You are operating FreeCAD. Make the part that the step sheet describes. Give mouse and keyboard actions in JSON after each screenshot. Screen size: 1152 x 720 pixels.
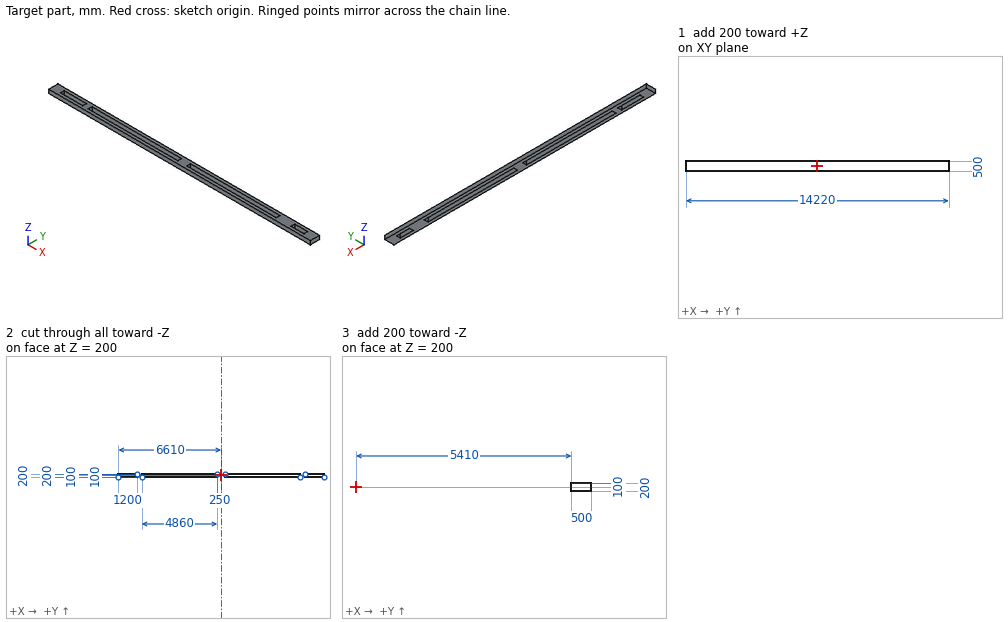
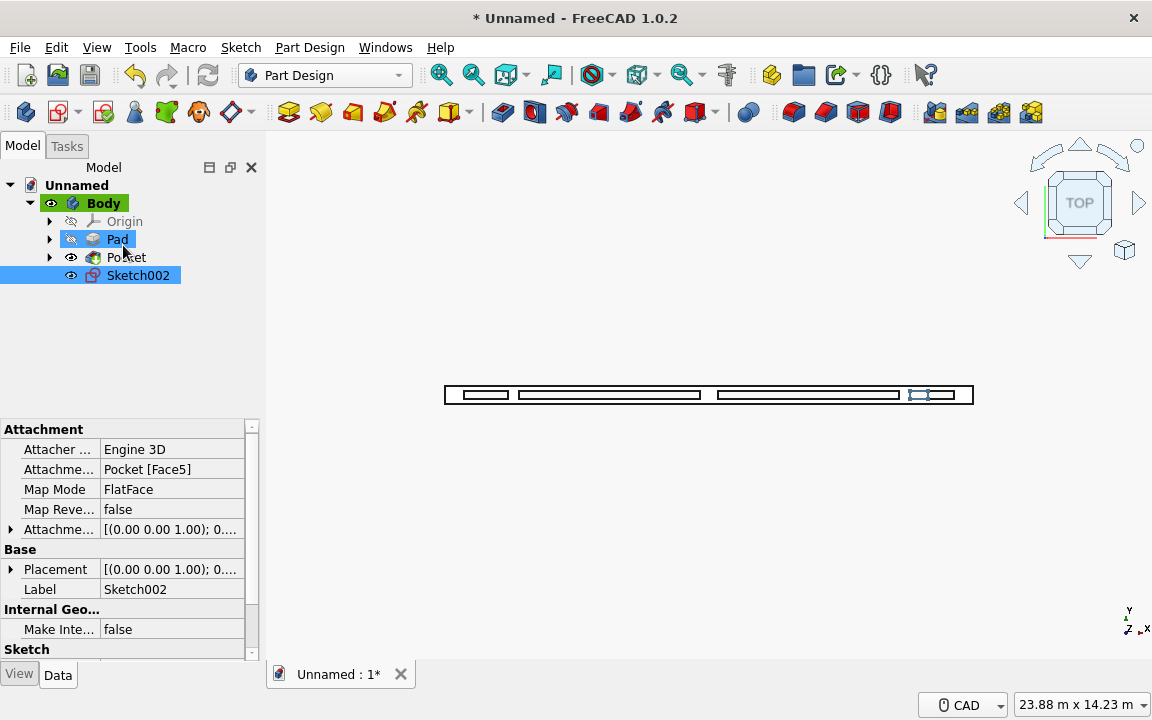
{"action": "left_click", "coordinate": [290, 112]}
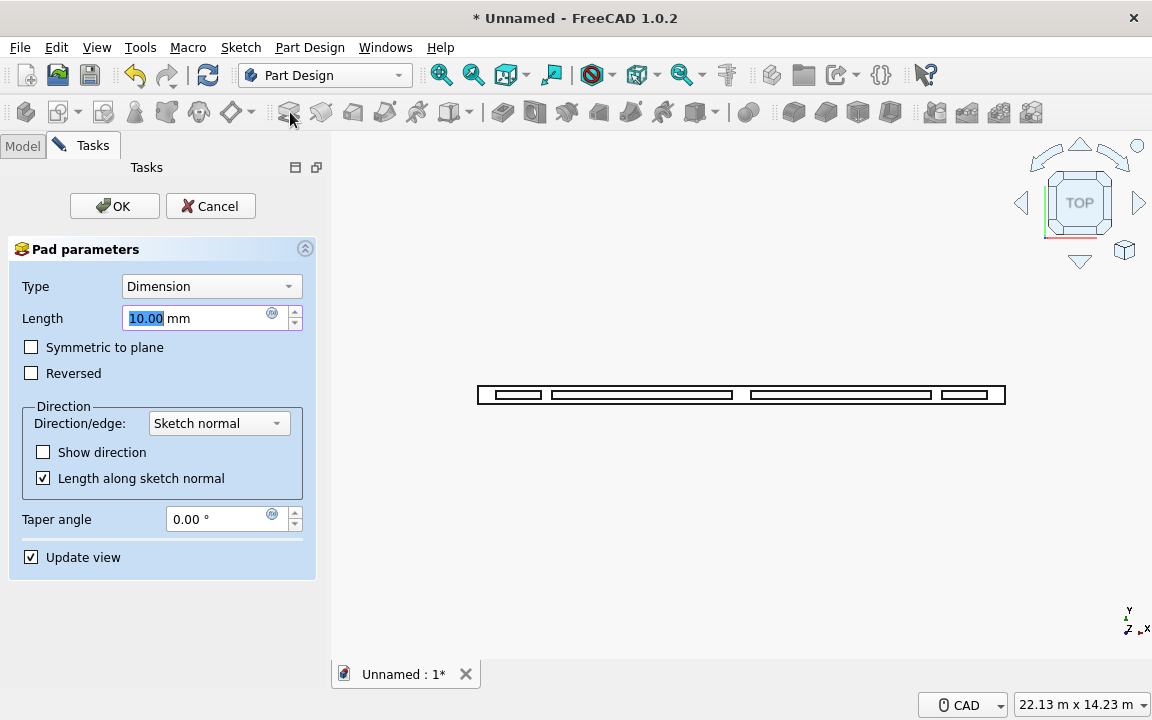
{"action": "type", "text": "200"}
{"action": "key", "text": "Tab"}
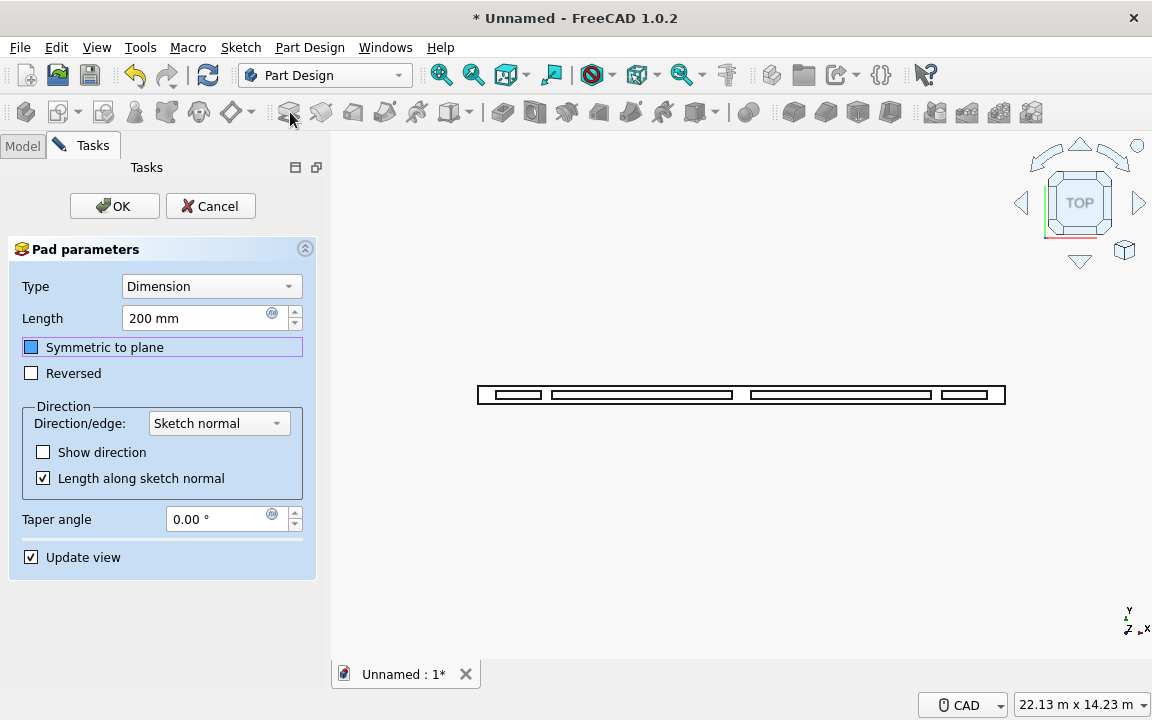
{"action": "left_click", "coordinate": [30, 373]}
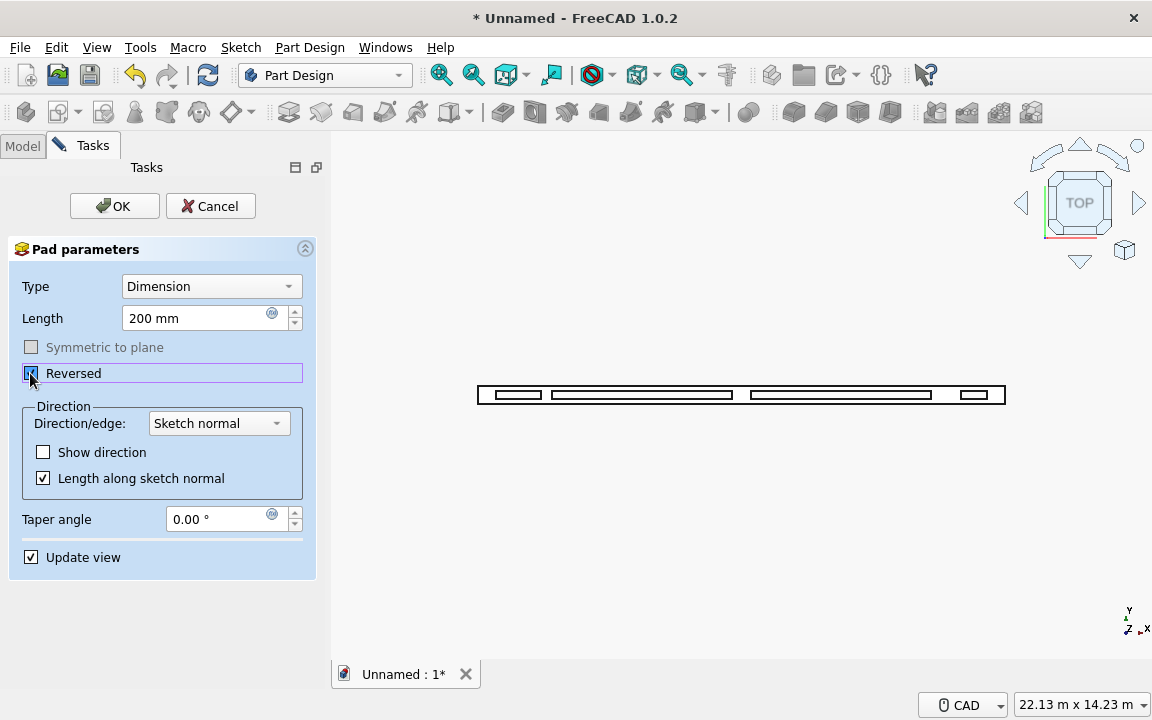
{"action": "left_click", "coordinate": [115, 206]}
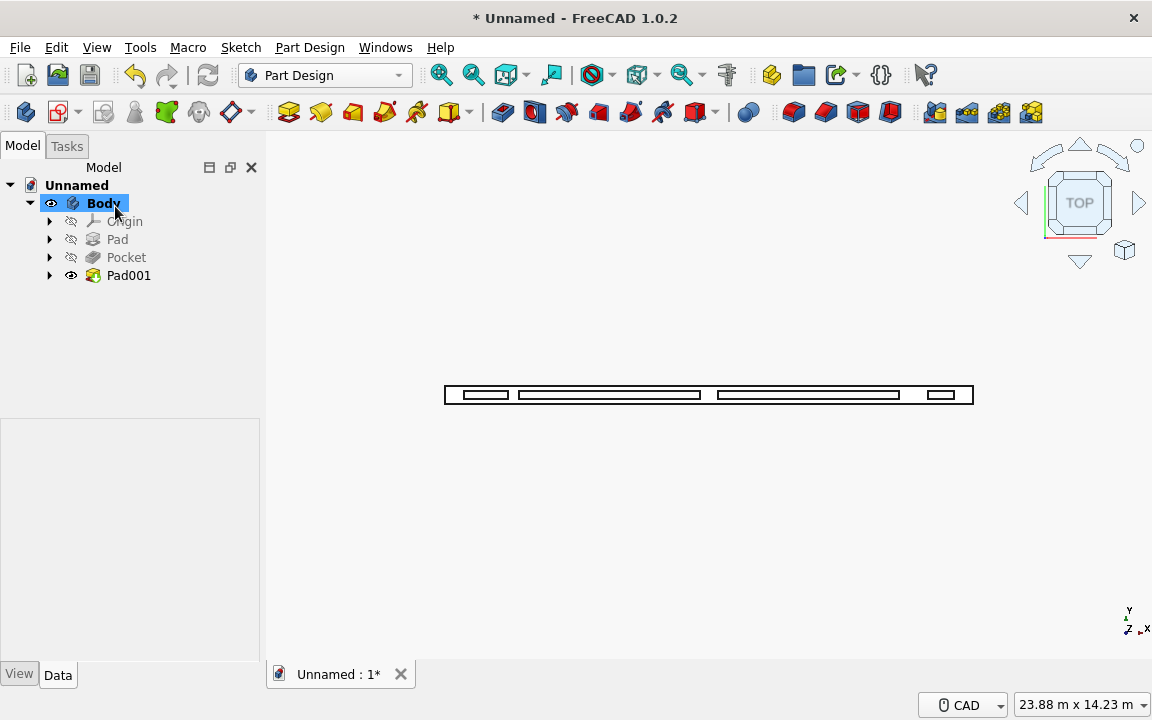
{"action": "key", "text": "0"}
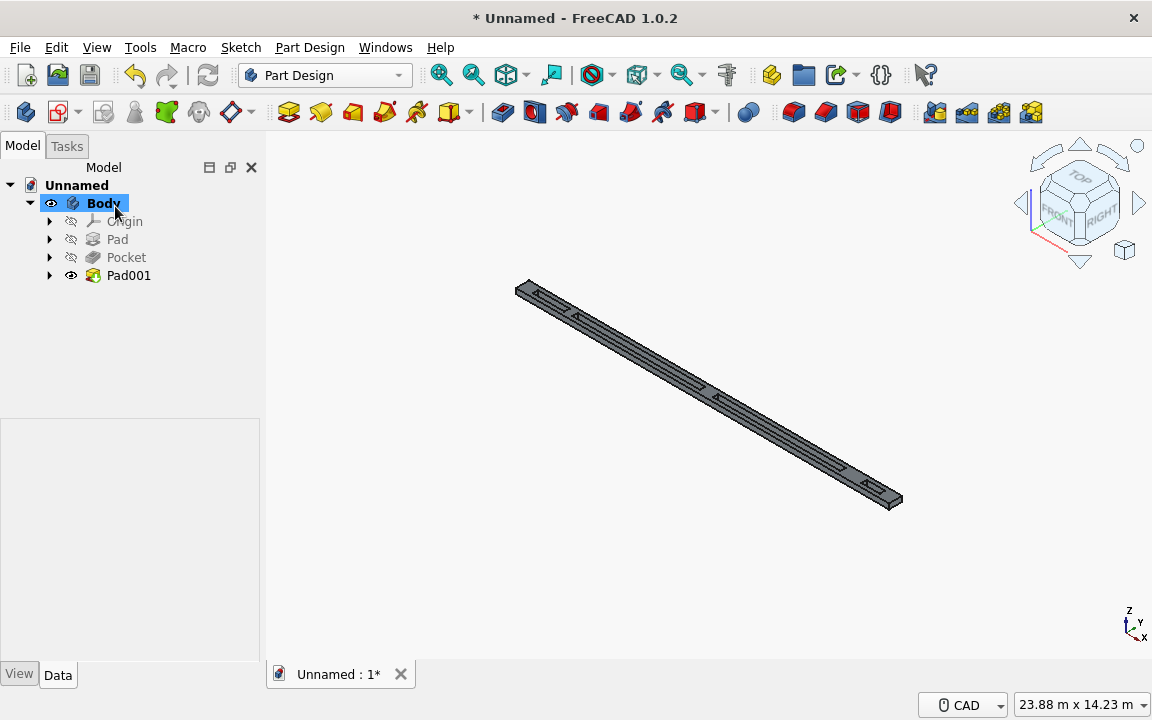
{"action": "left_click", "coordinate": [442, 76]}